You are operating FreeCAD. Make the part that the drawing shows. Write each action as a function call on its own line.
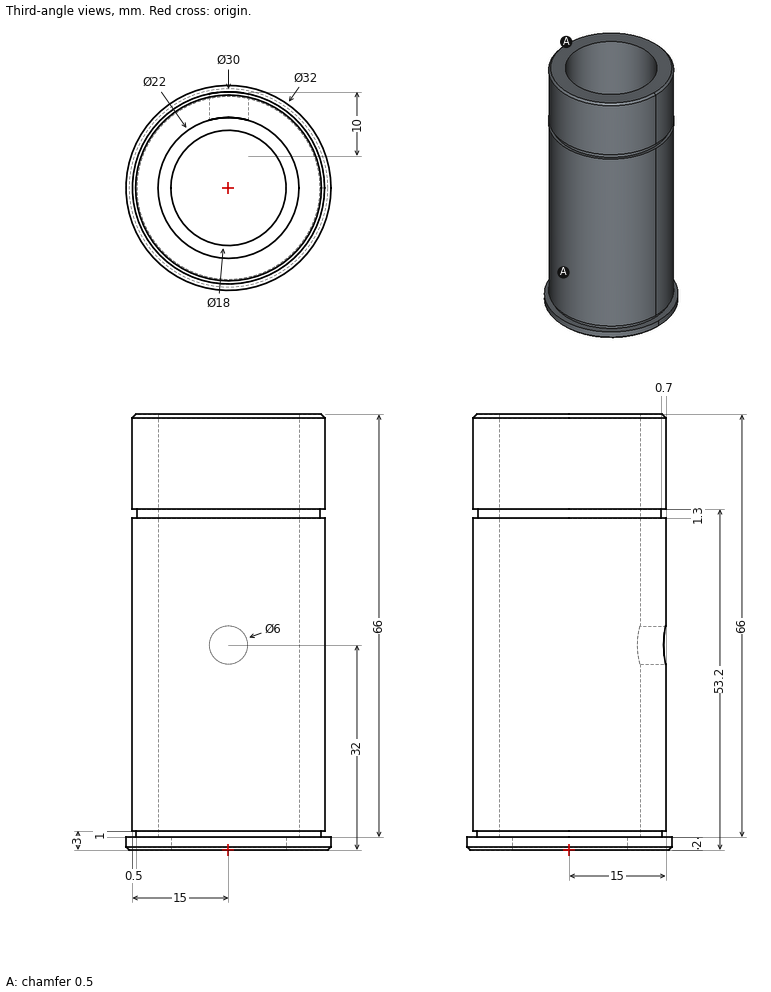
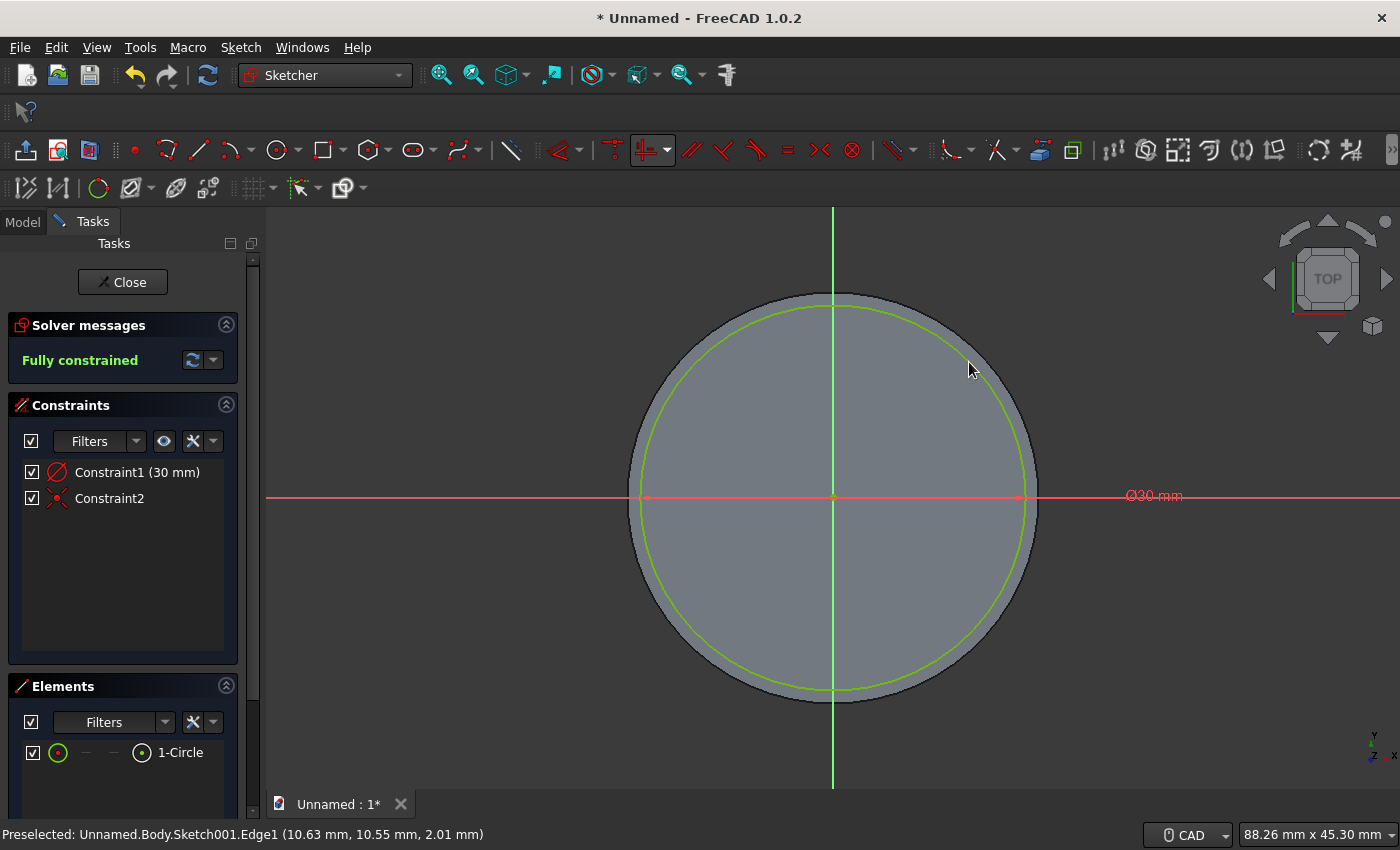
click(123, 282)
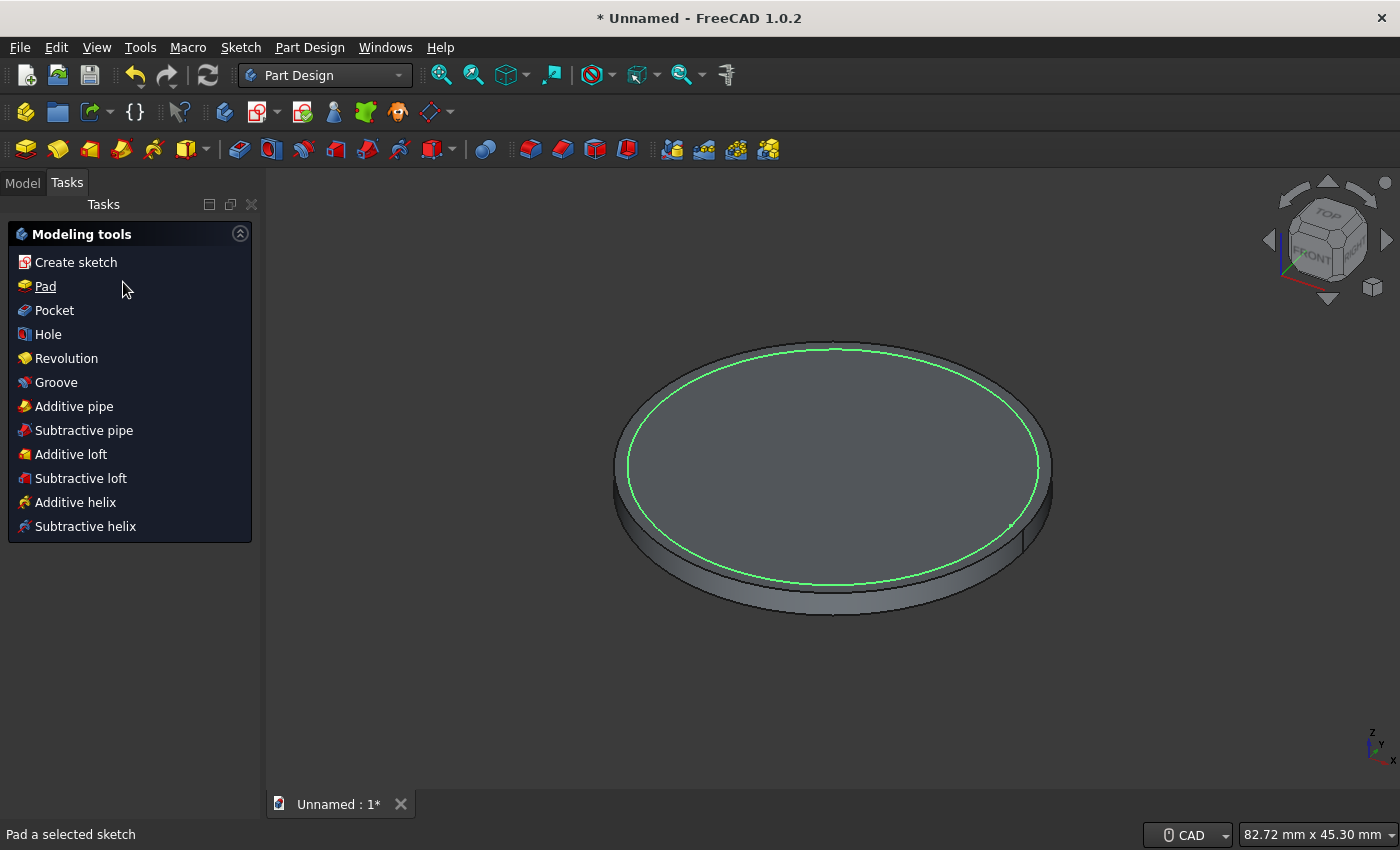
click(26, 150)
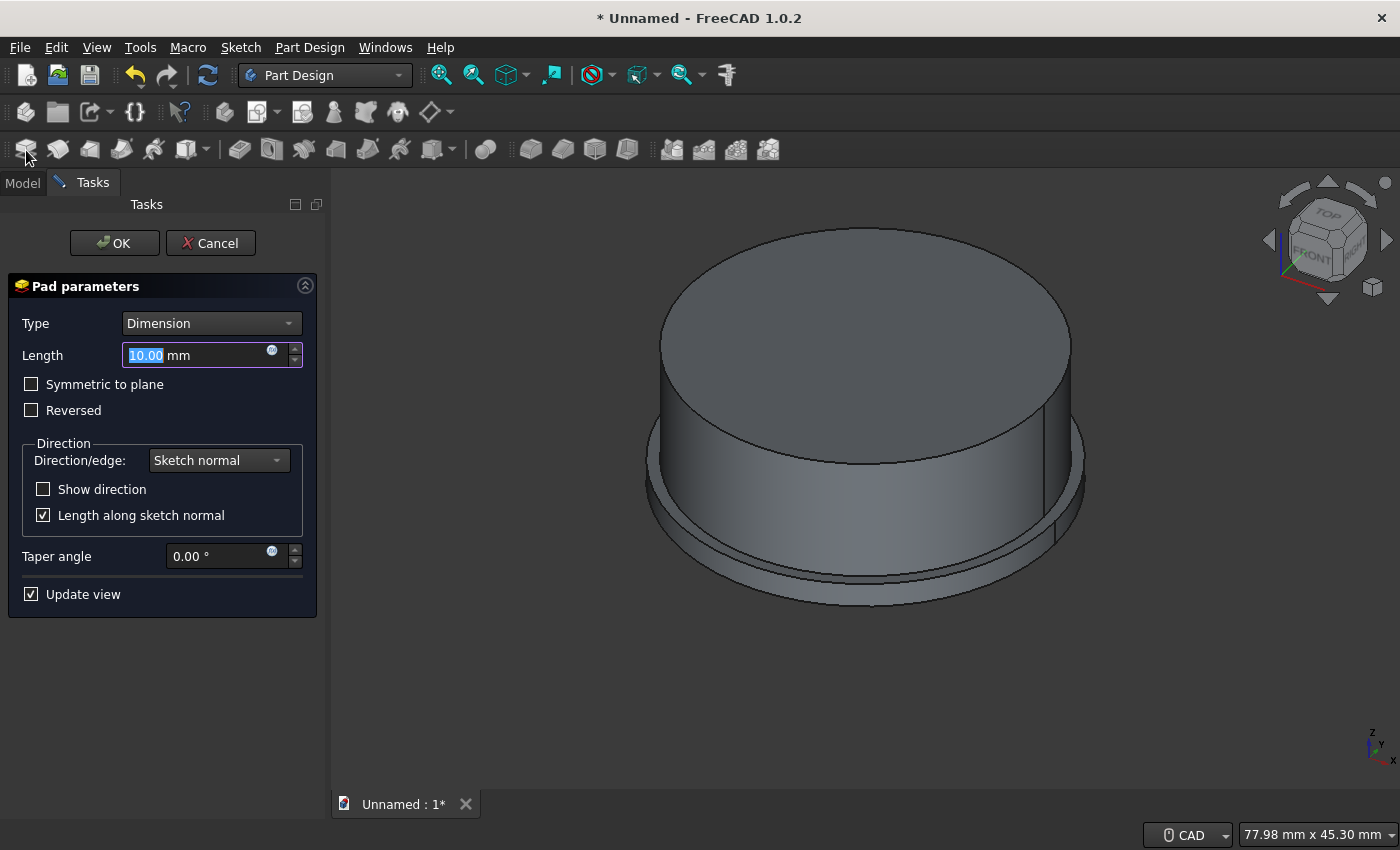
text(66)
key(Tab)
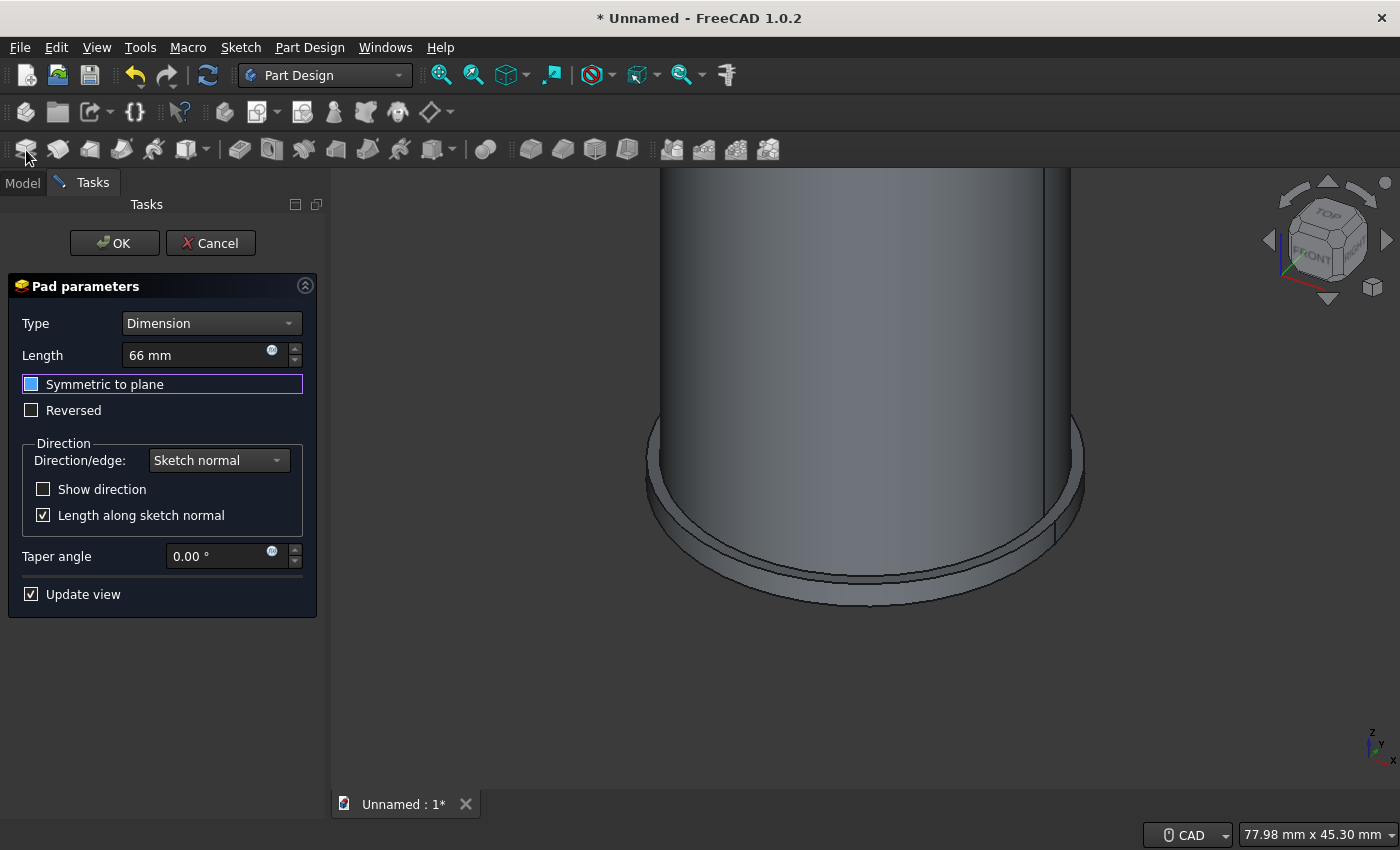
click(115, 243)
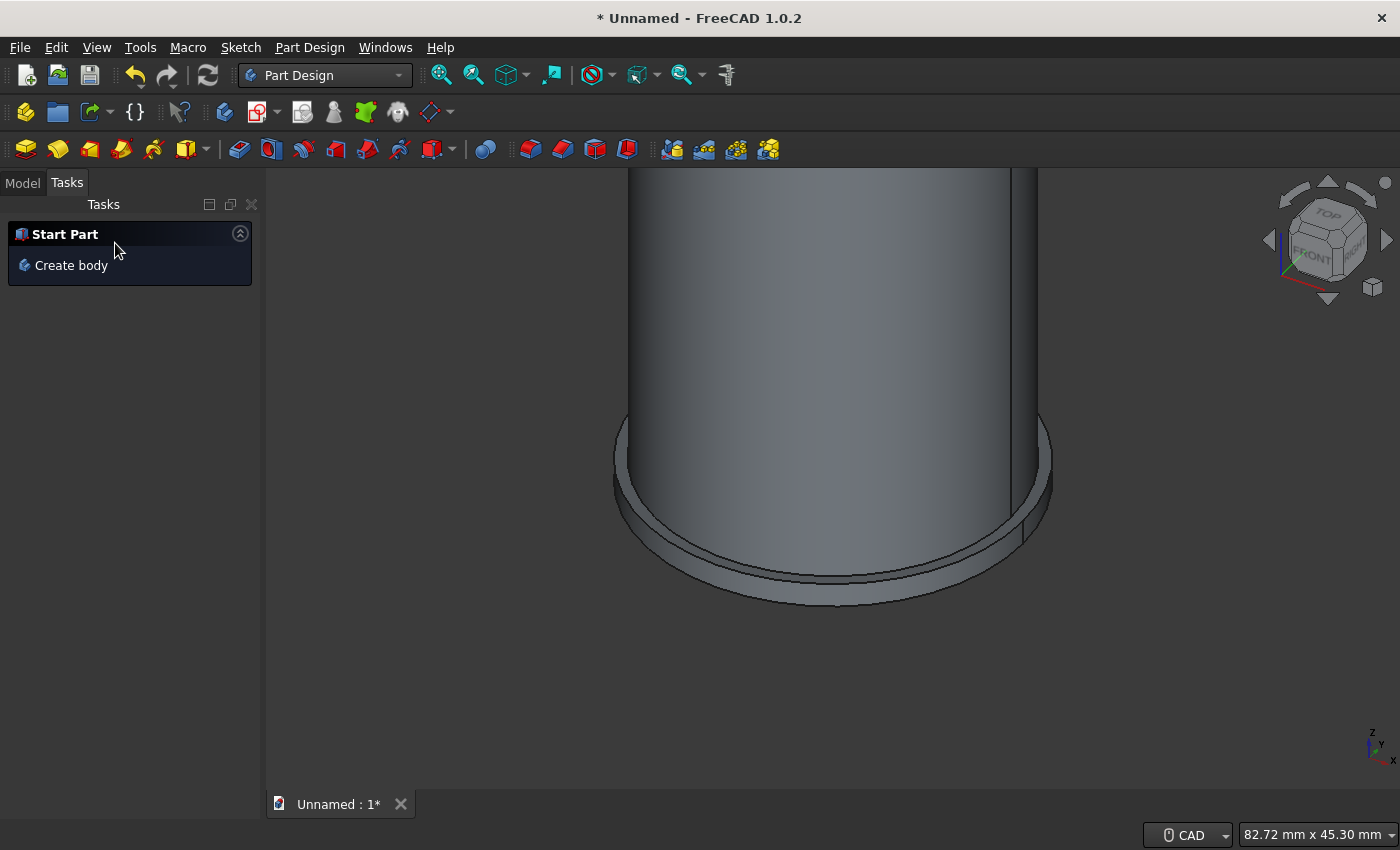
click(442, 76)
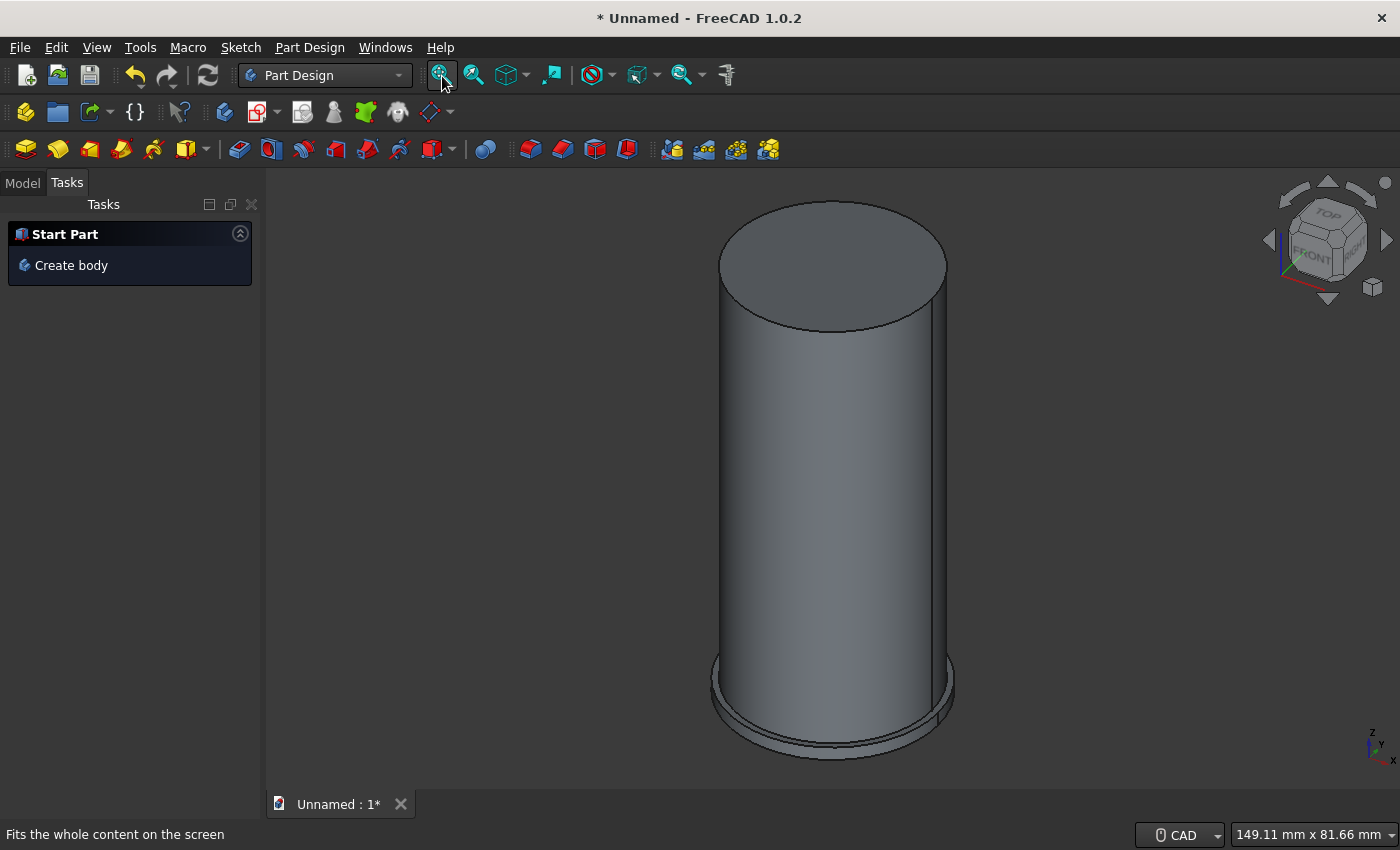
click(258, 112)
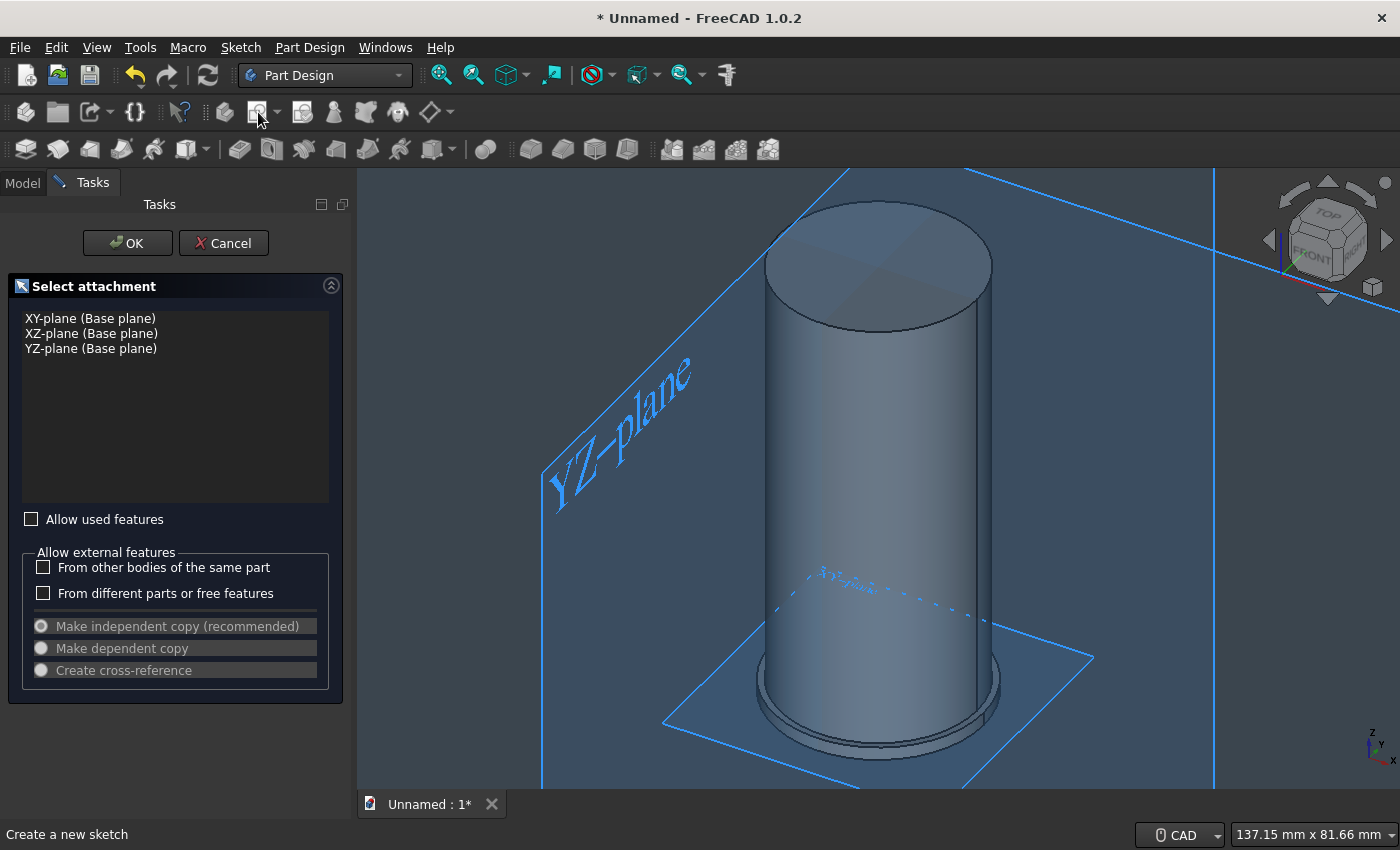
click(82, 318)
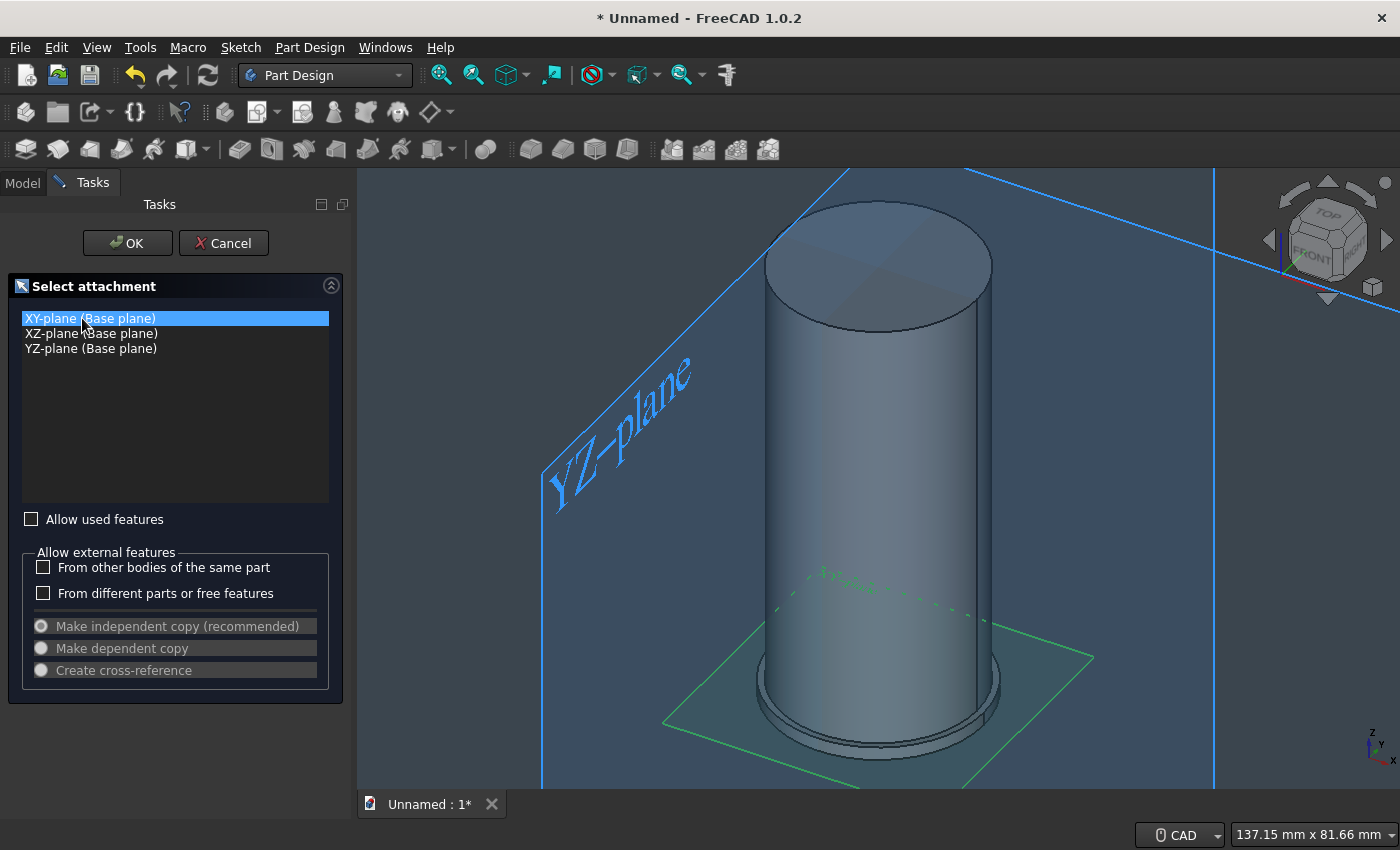
click(128, 243)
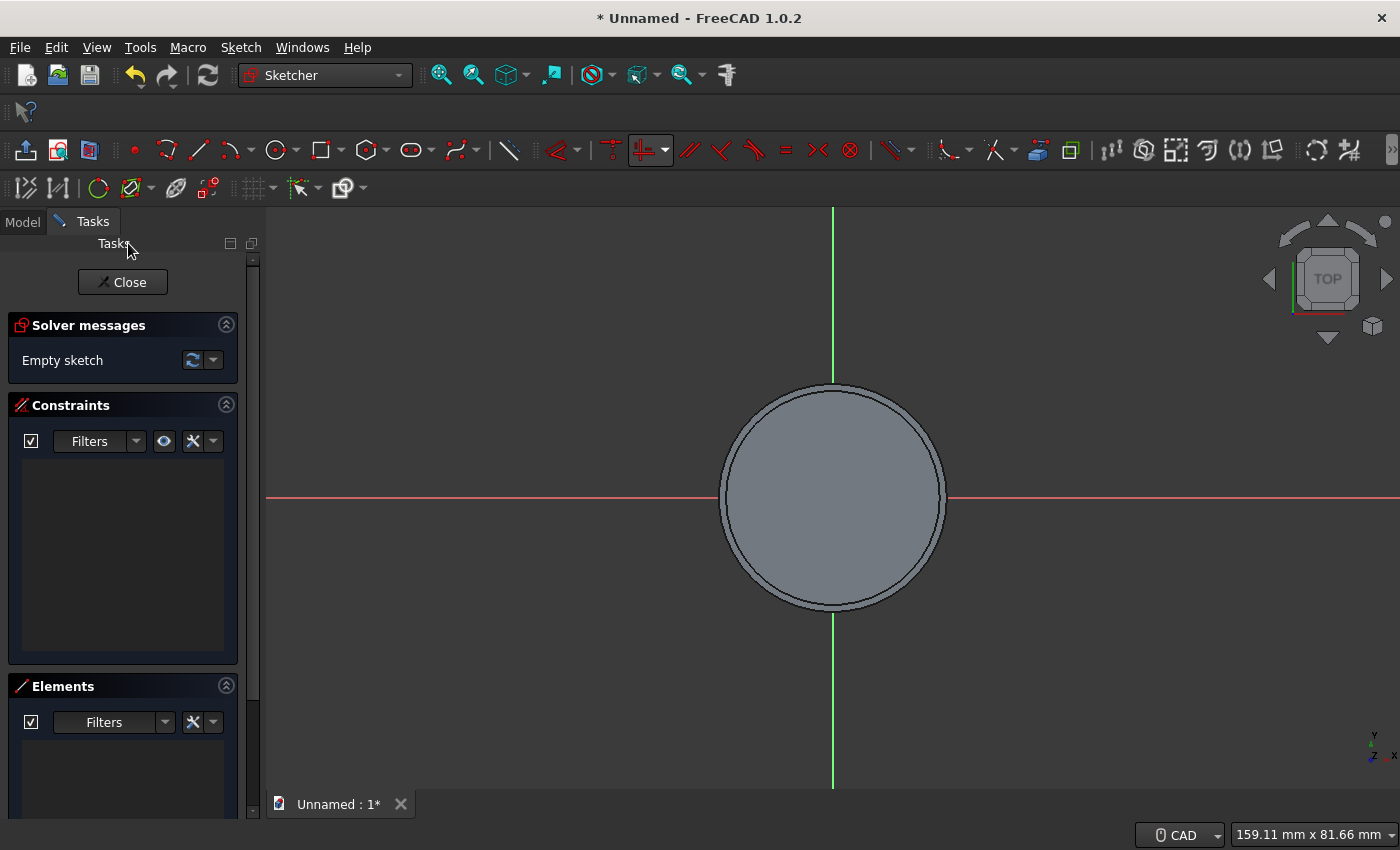
key(q)
key(s)